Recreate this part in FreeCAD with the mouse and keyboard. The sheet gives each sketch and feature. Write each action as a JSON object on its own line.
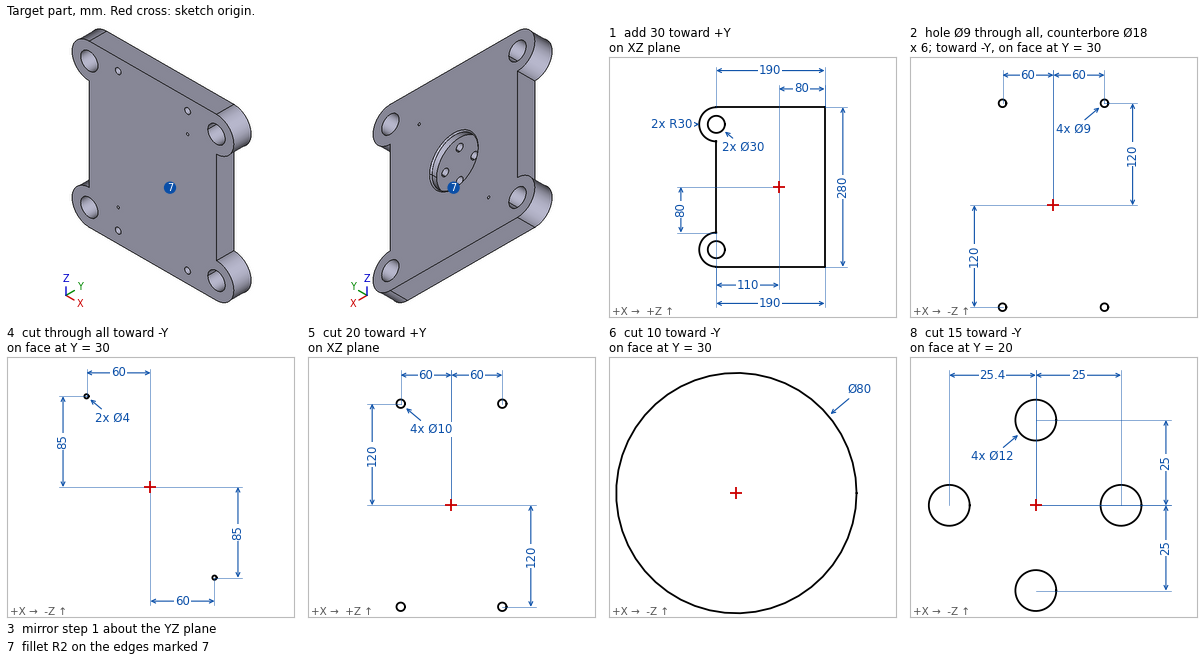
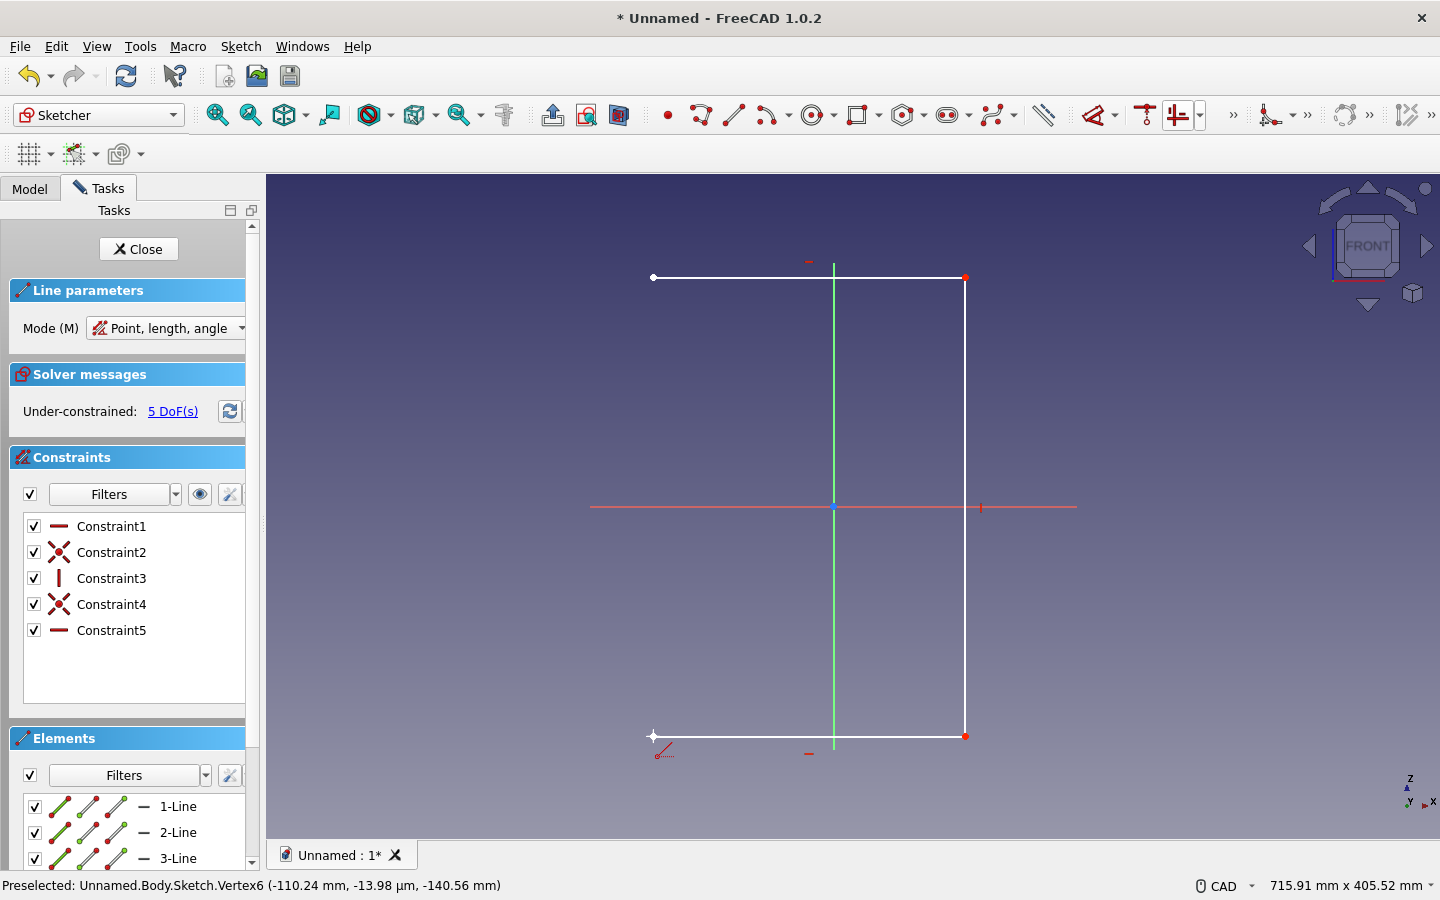
{"action": "left_click", "coordinate": [653, 638]}
{"action": "left_click", "coordinate": [653, 375]}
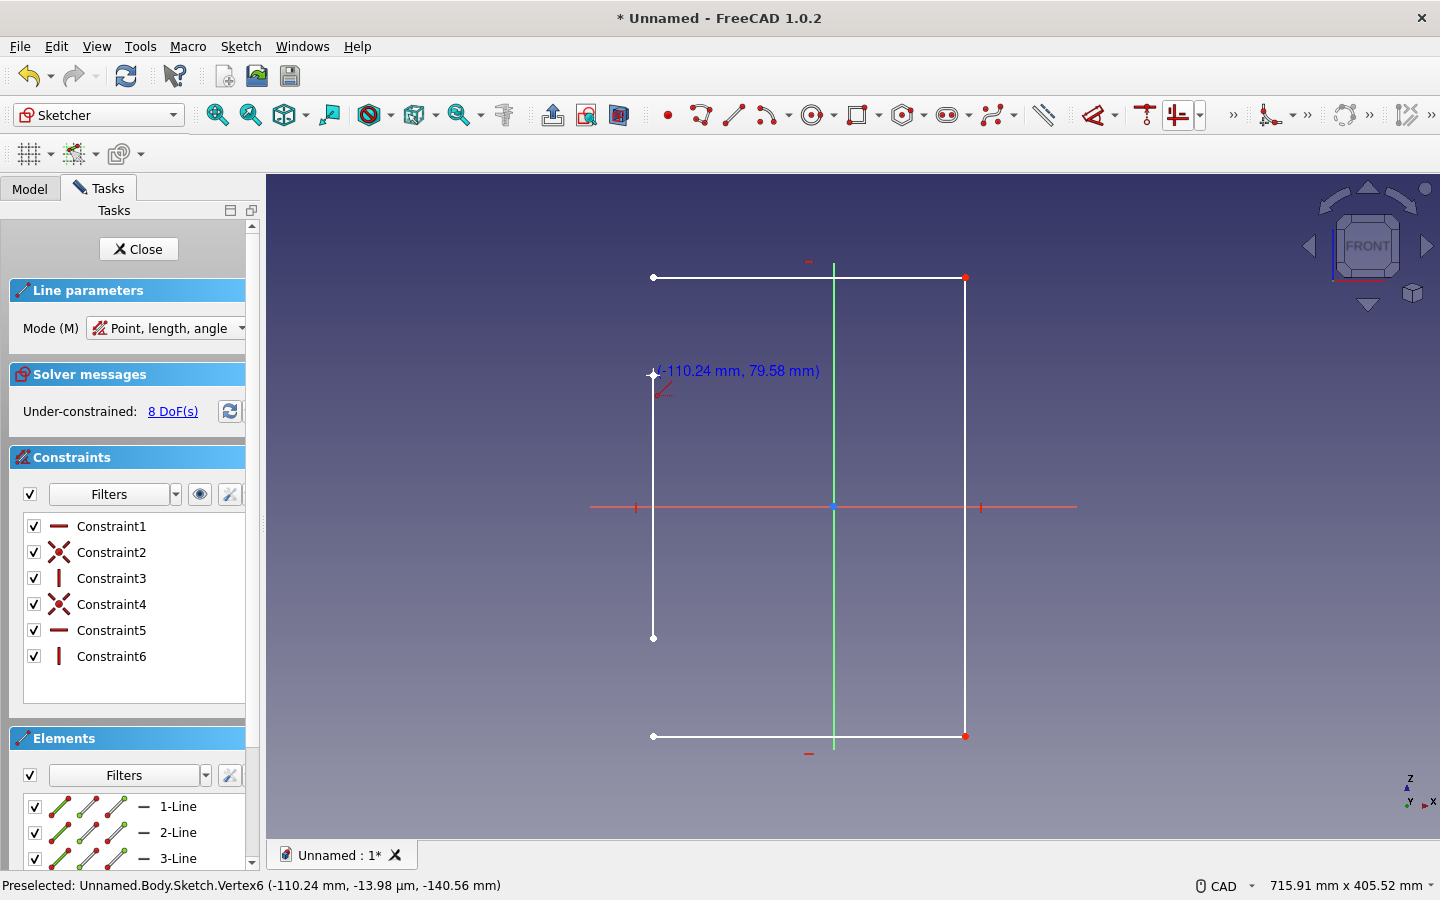
{"action": "left_click", "coordinate": [788, 116]}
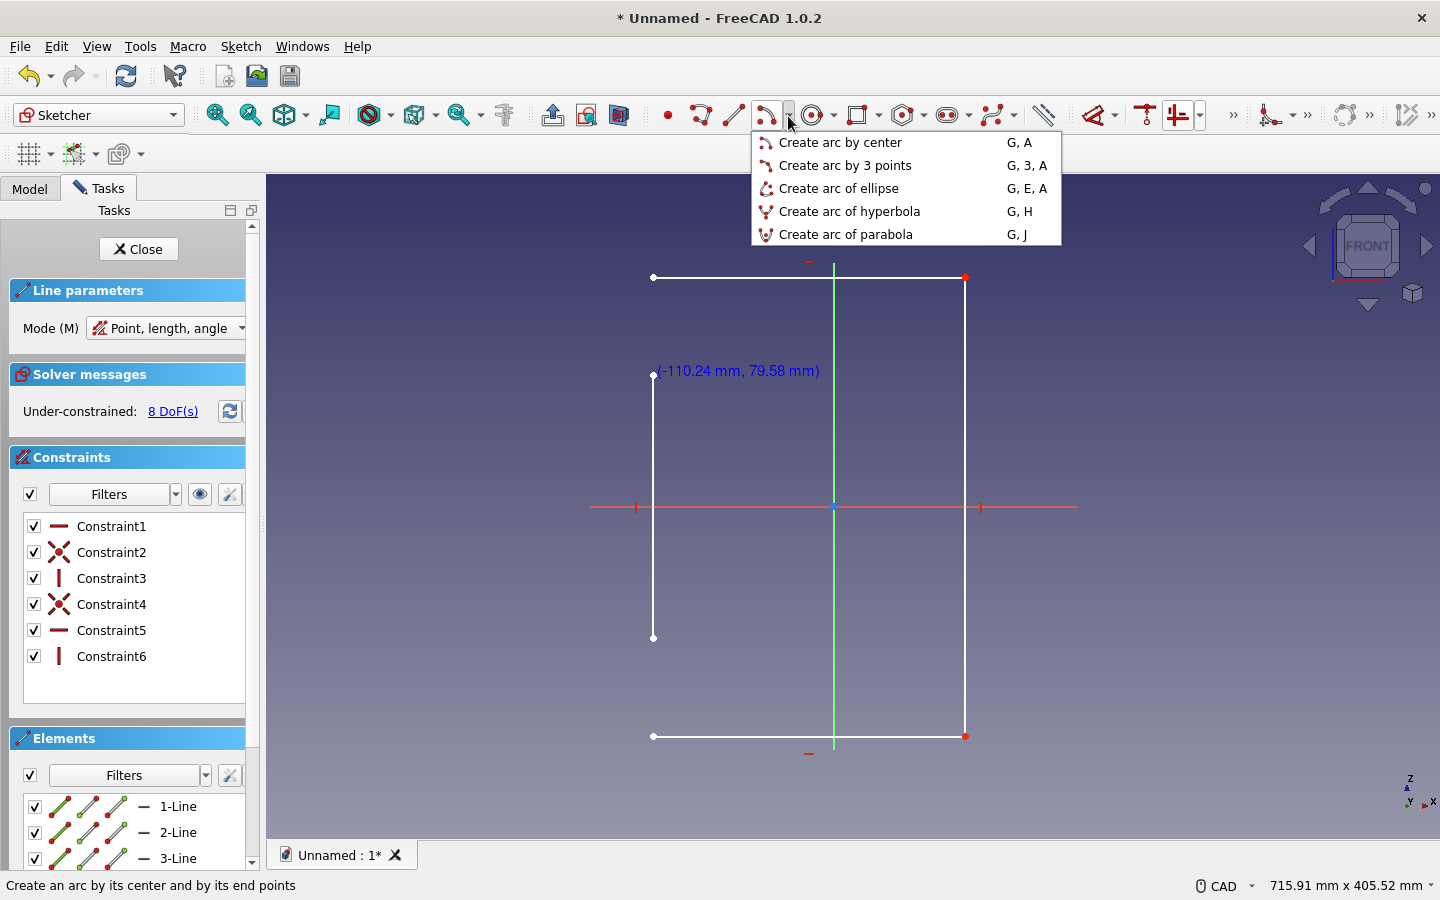
{"action": "left_click", "coordinate": [906, 166]}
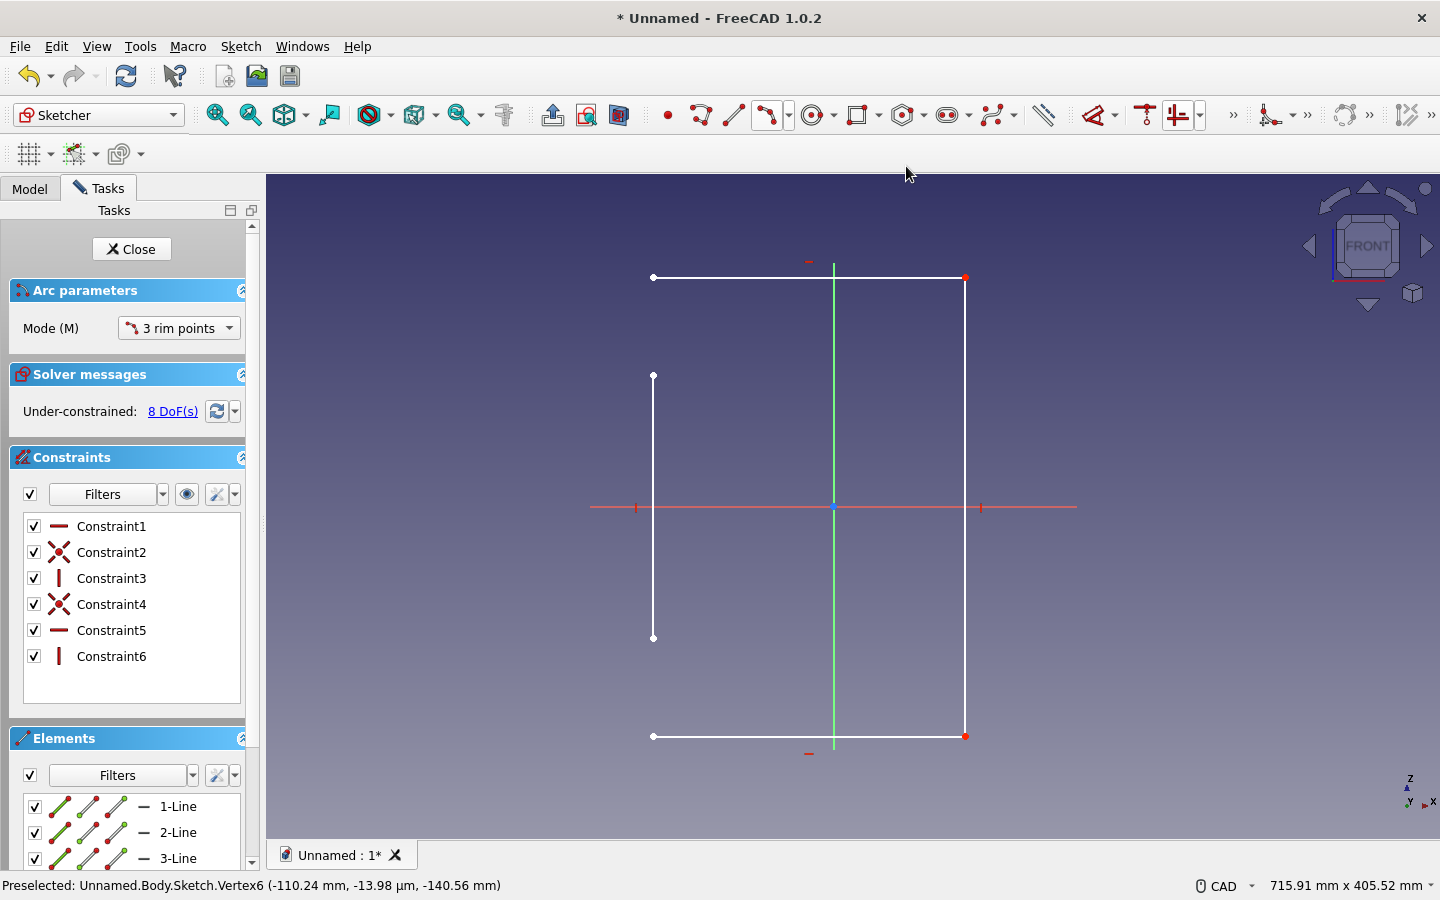
{"action": "left_click", "coordinate": [653, 737]}
{"action": "left_click", "coordinate": [653, 639]}
{"action": "left_click", "coordinate": [604, 687]}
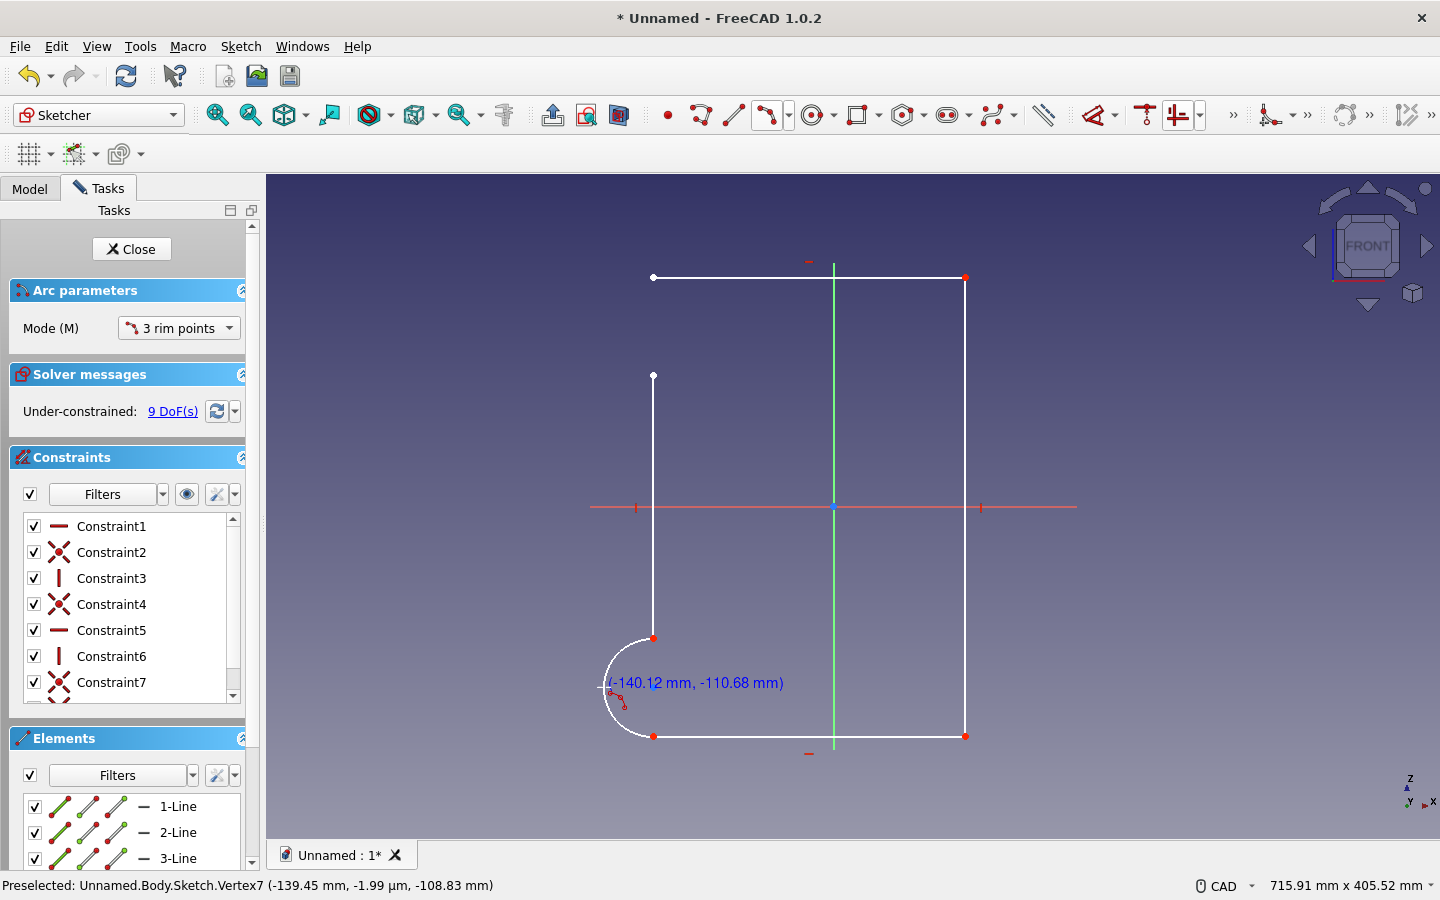
{"action": "left_click", "coordinate": [653, 376]}
{"action": "left_click", "coordinate": [653, 278]}
{"action": "left_click", "coordinate": [604, 326]}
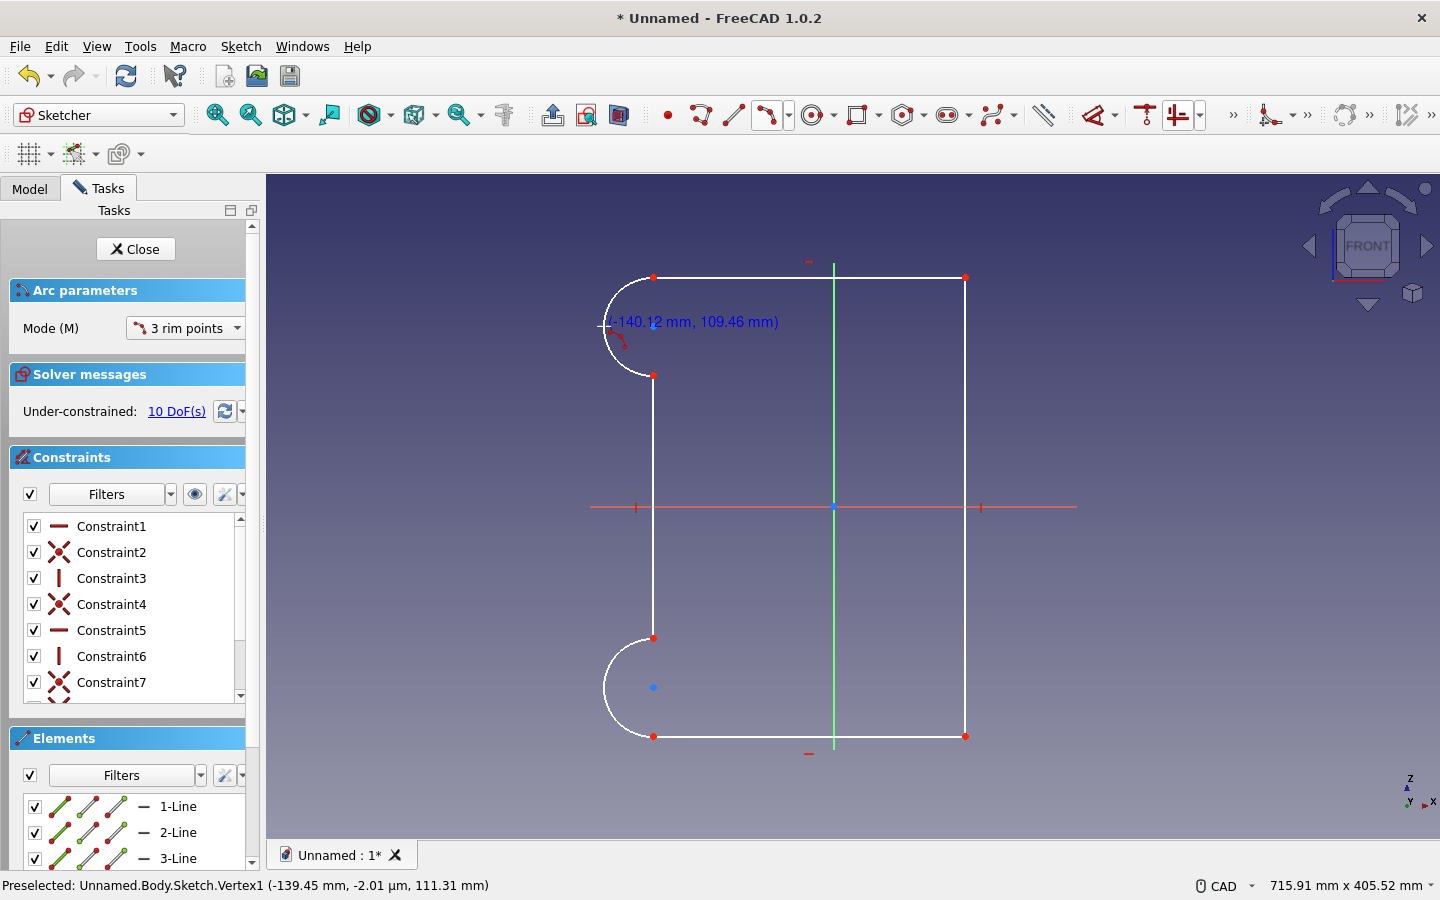
{"action": "left_click", "coordinate": [812, 116]}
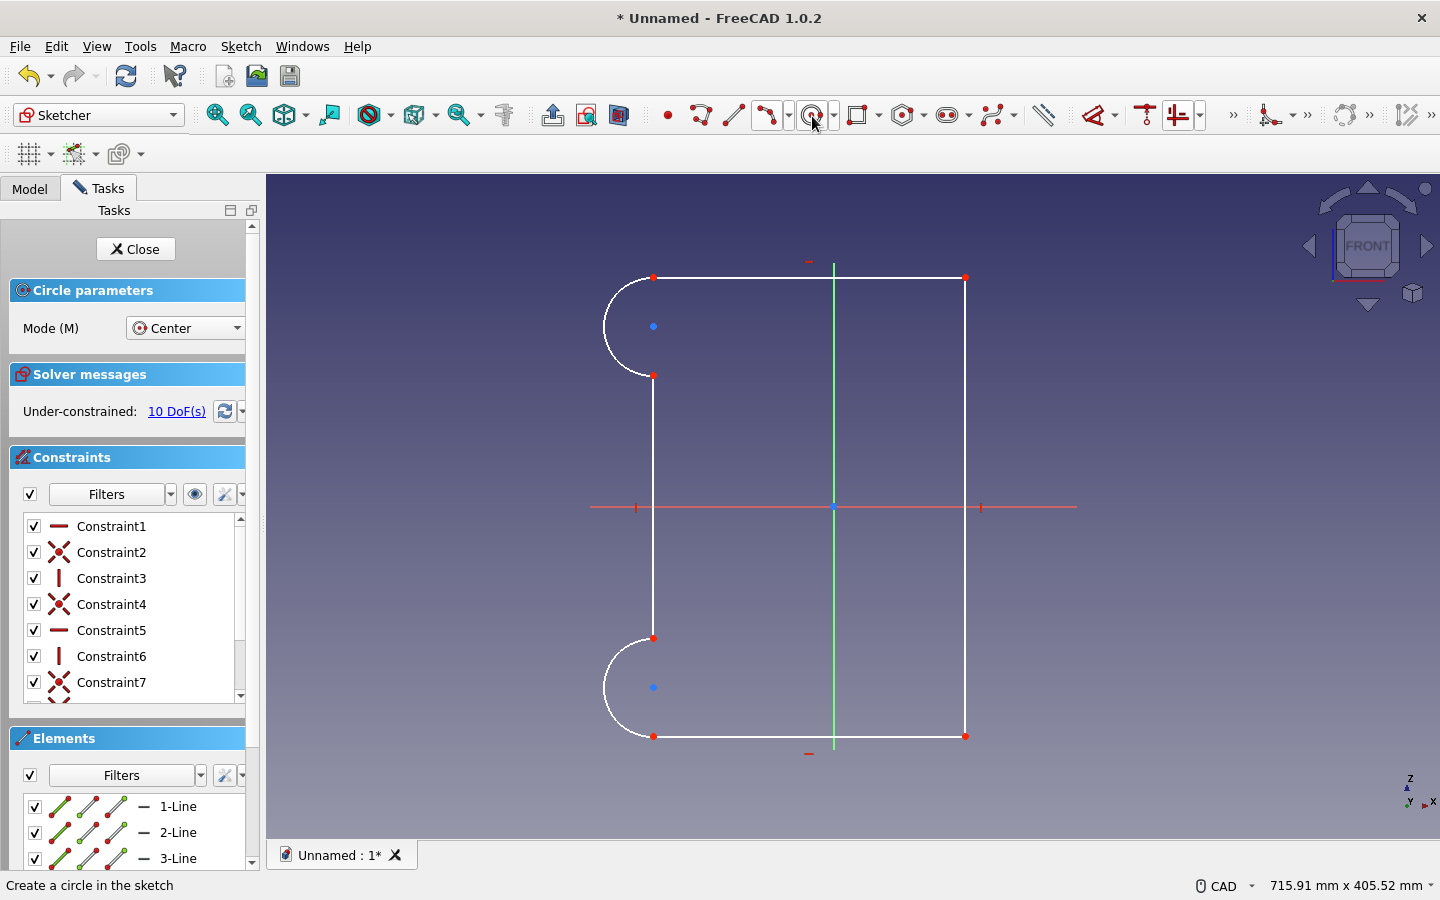
{"action": "left_click", "coordinate": [653, 326]}
{"action": "mouse_move", "coordinate": [671, 309]}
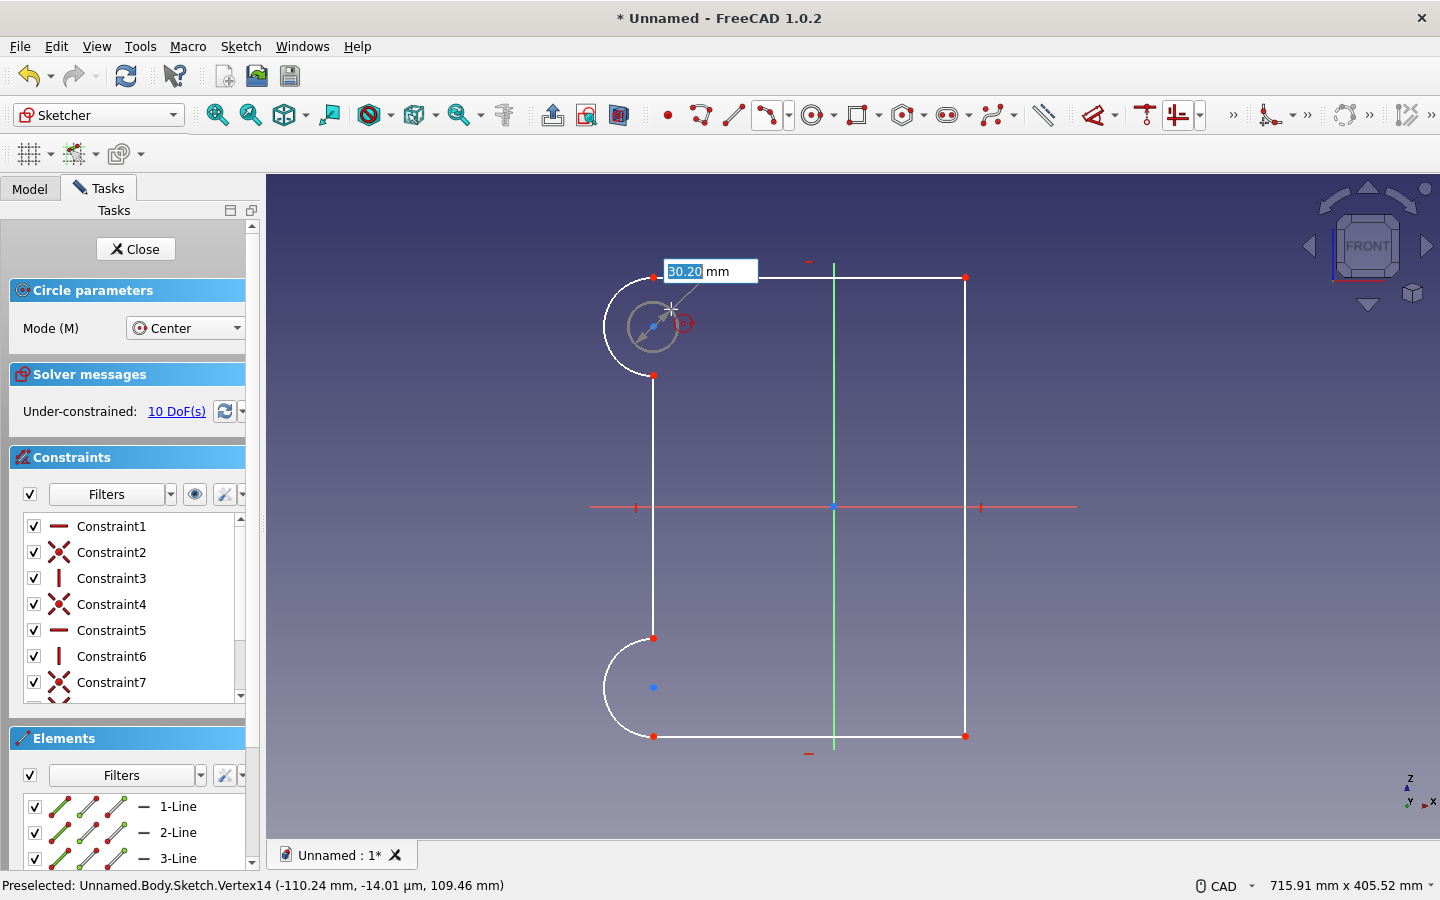
{"action": "type", "text": "30"}
{"action": "key", "text": "Return"}